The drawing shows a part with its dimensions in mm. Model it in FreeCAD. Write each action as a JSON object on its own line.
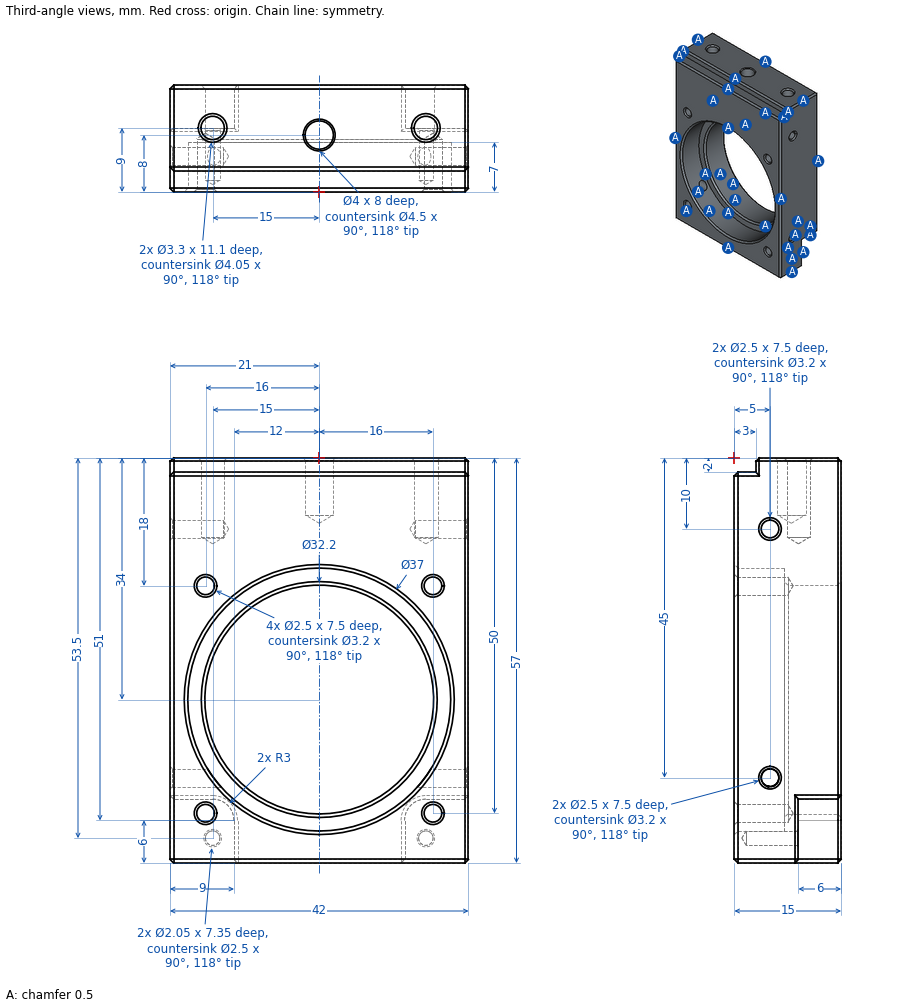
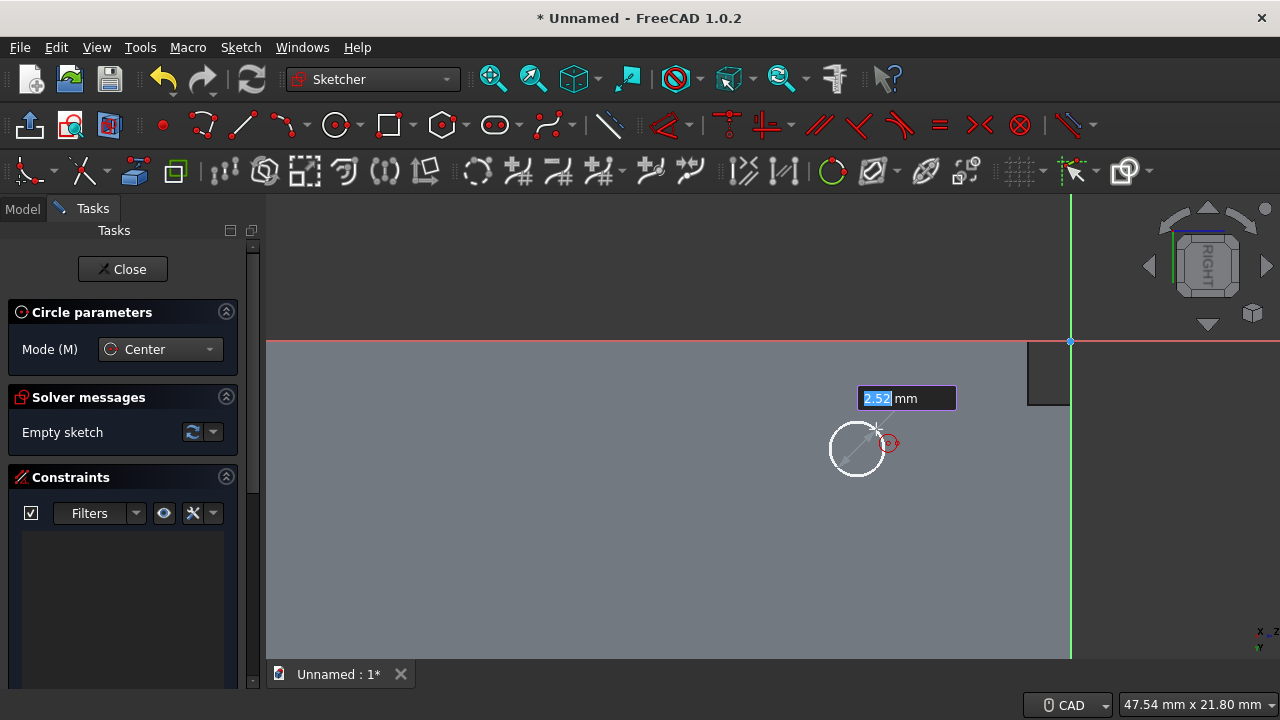
{"action": "type", "text": "2.5"}
{"action": "key", "text": "Return"}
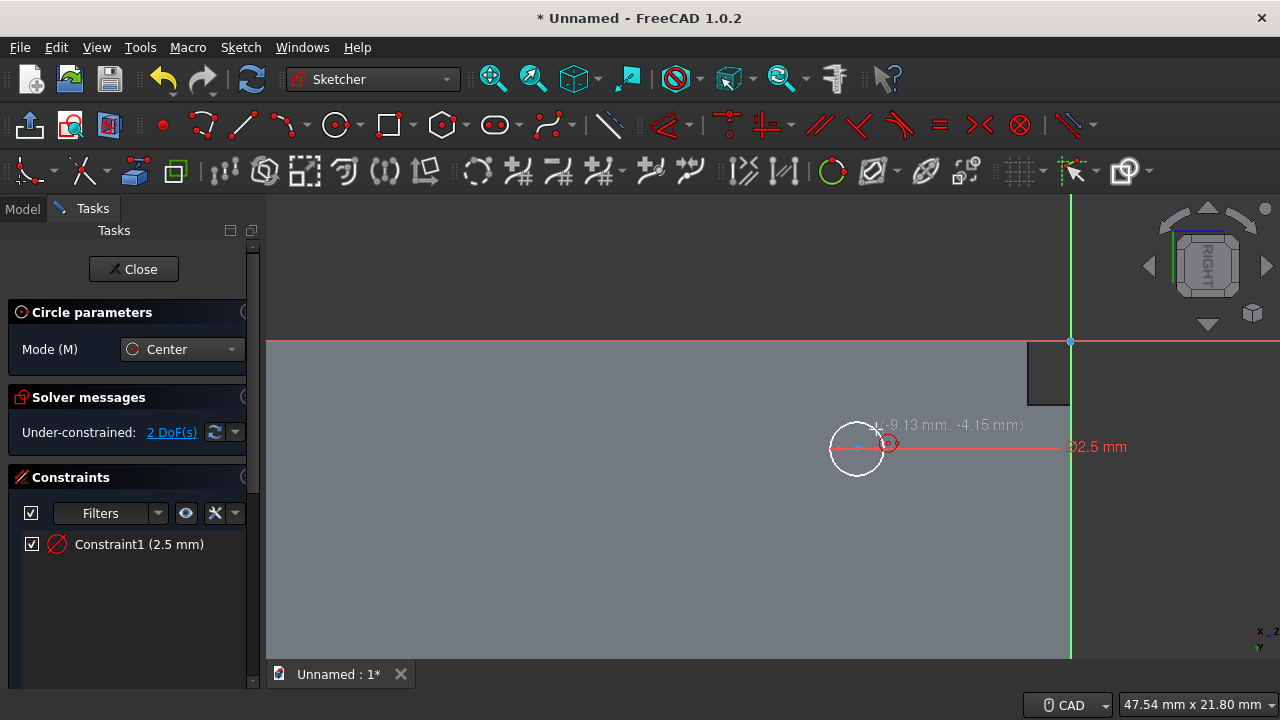
{"action": "scroll", "coordinate": [859, 449], "scroll_direction": "down", "scroll_amount": 3}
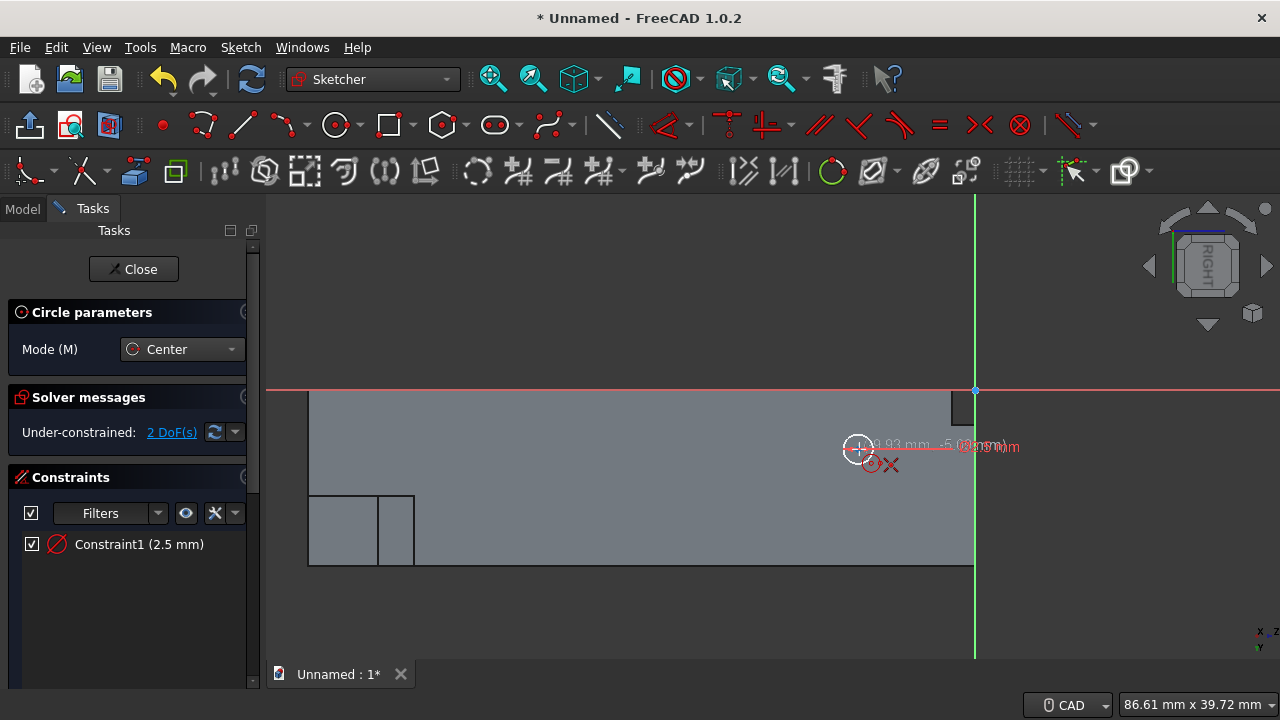
{"action": "scroll", "coordinate": [449, 449], "scroll_direction": "up", "scroll_amount": 3}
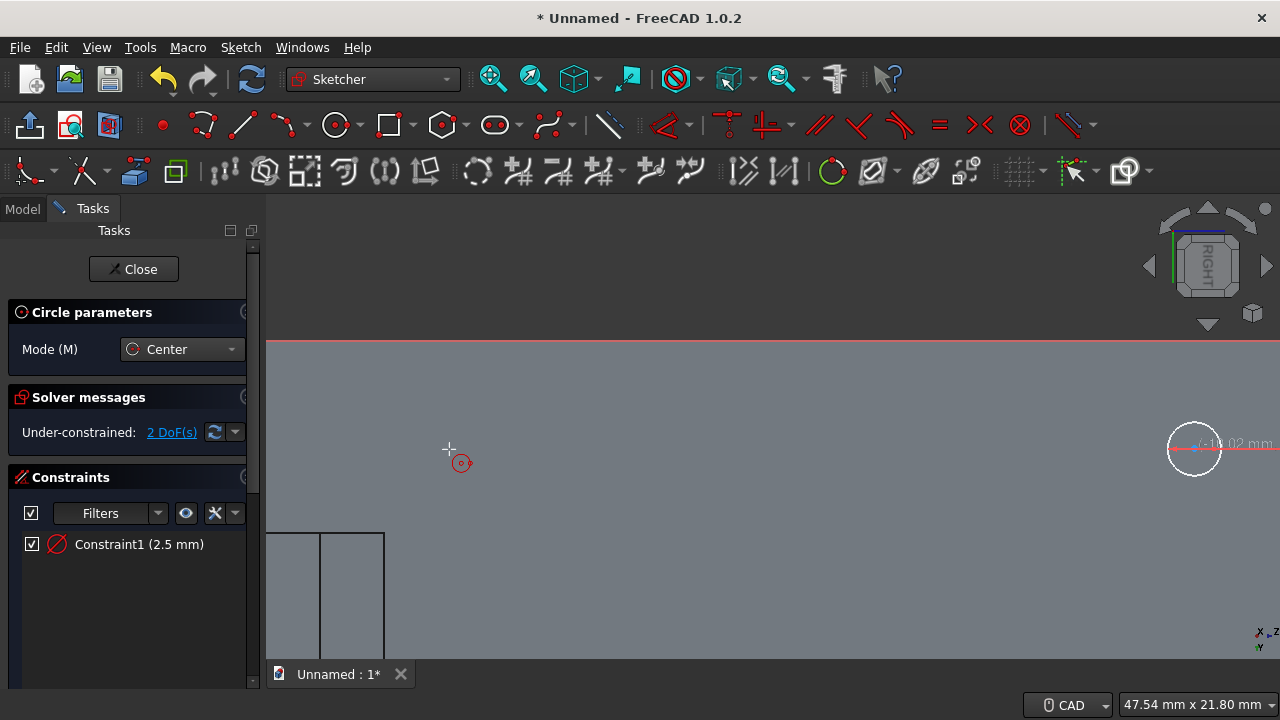
{"action": "left_click", "coordinate": [448, 448]}
{"action": "mouse_move", "coordinate": [467, 429]}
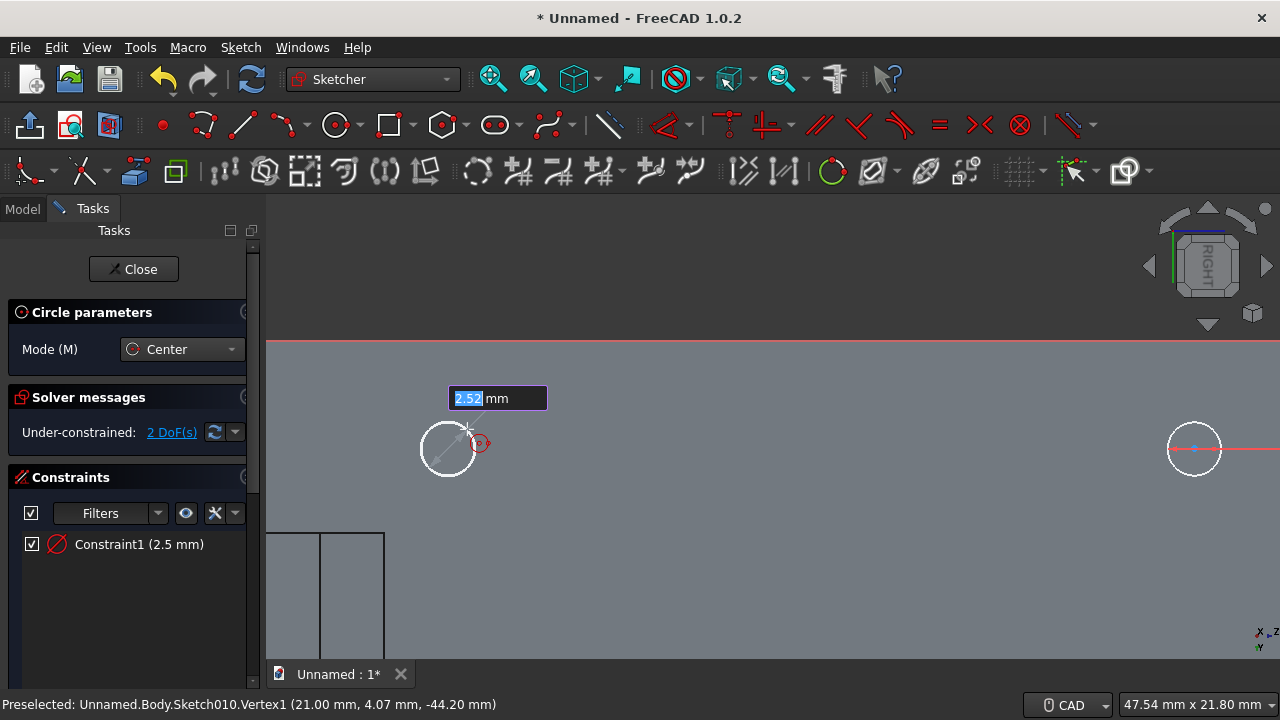
{"action": "type", "text": "2.5"}
{"action": "key", "text": "Return"}
{"action": "key", "text": "Escape"}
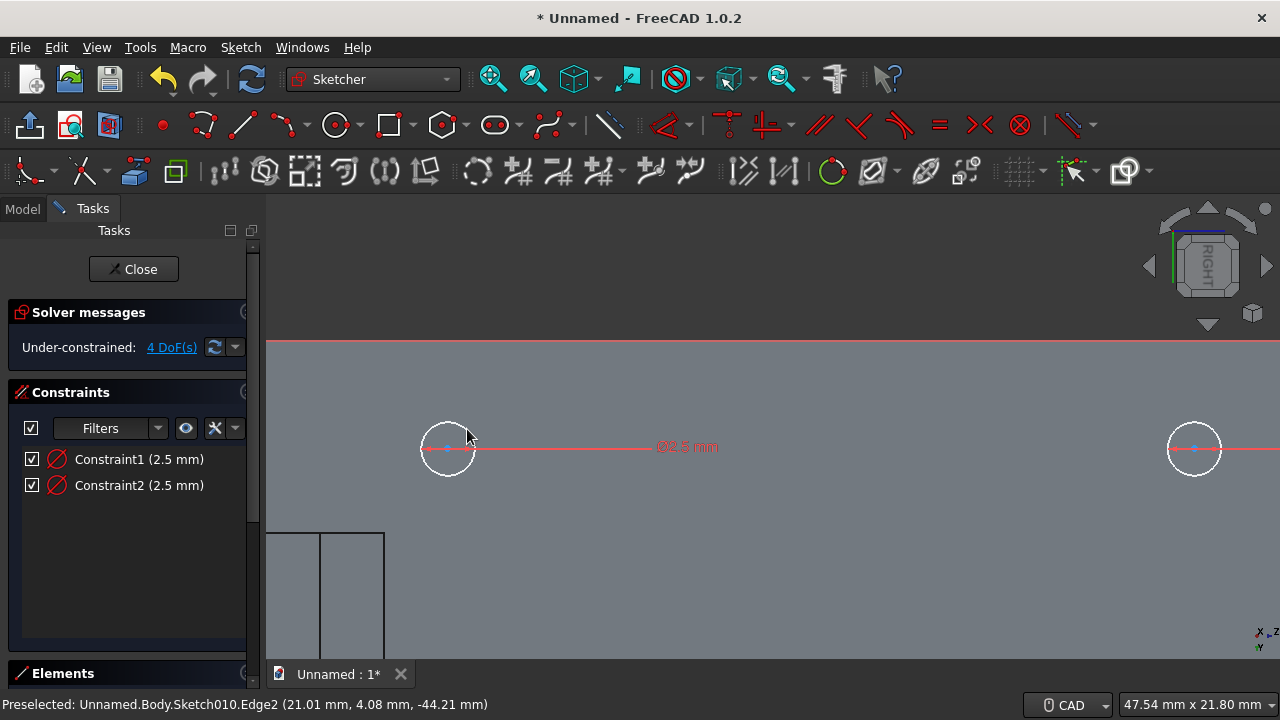
{"action": "key", "text": "d"}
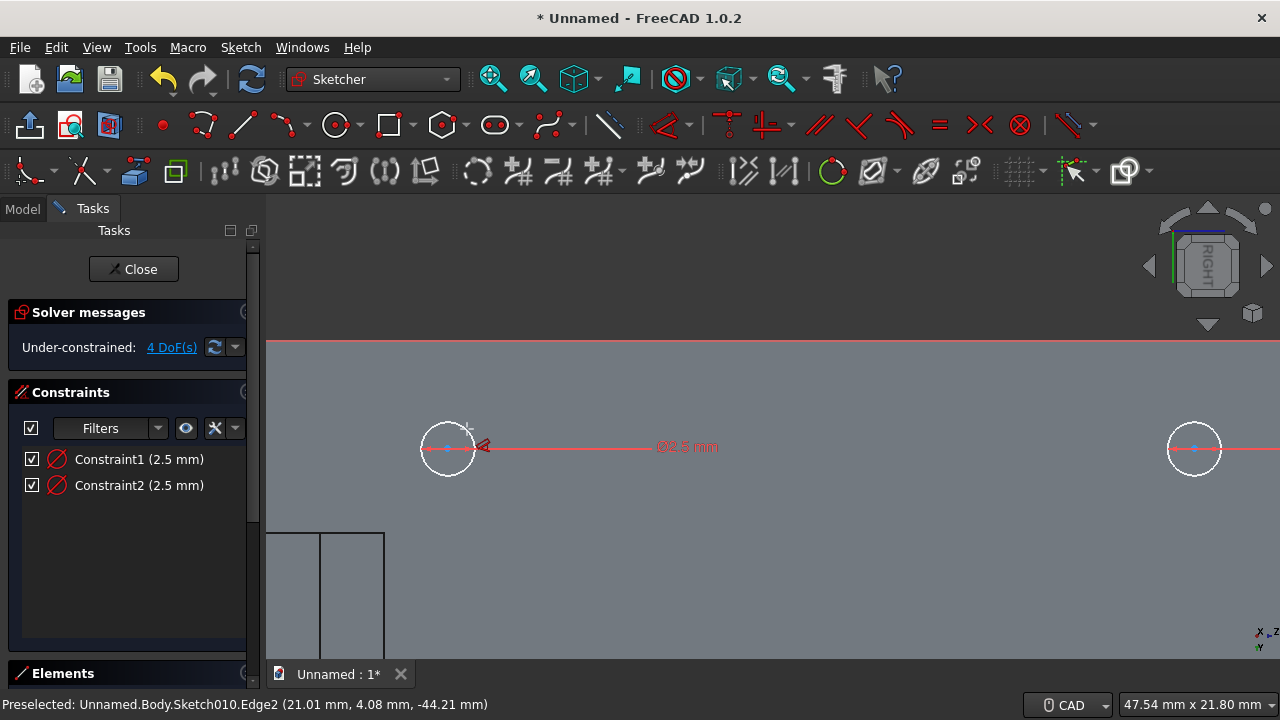
{"action": "scroll", "coordinate": [449, 449], "scroll_direction": "down", "scroll_amount": 3}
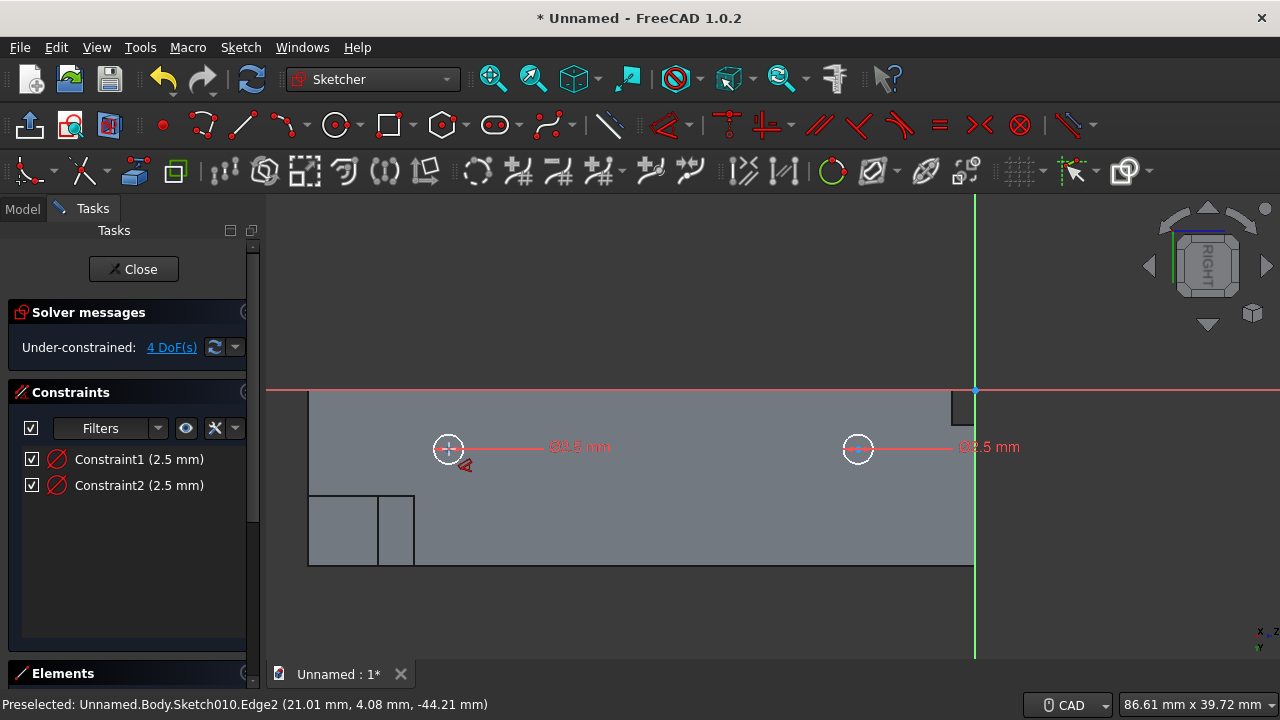
{"action": "left_click", "coordinate": [858, 449]}
{"action": "left_click", "coordinate": [1009, 420]}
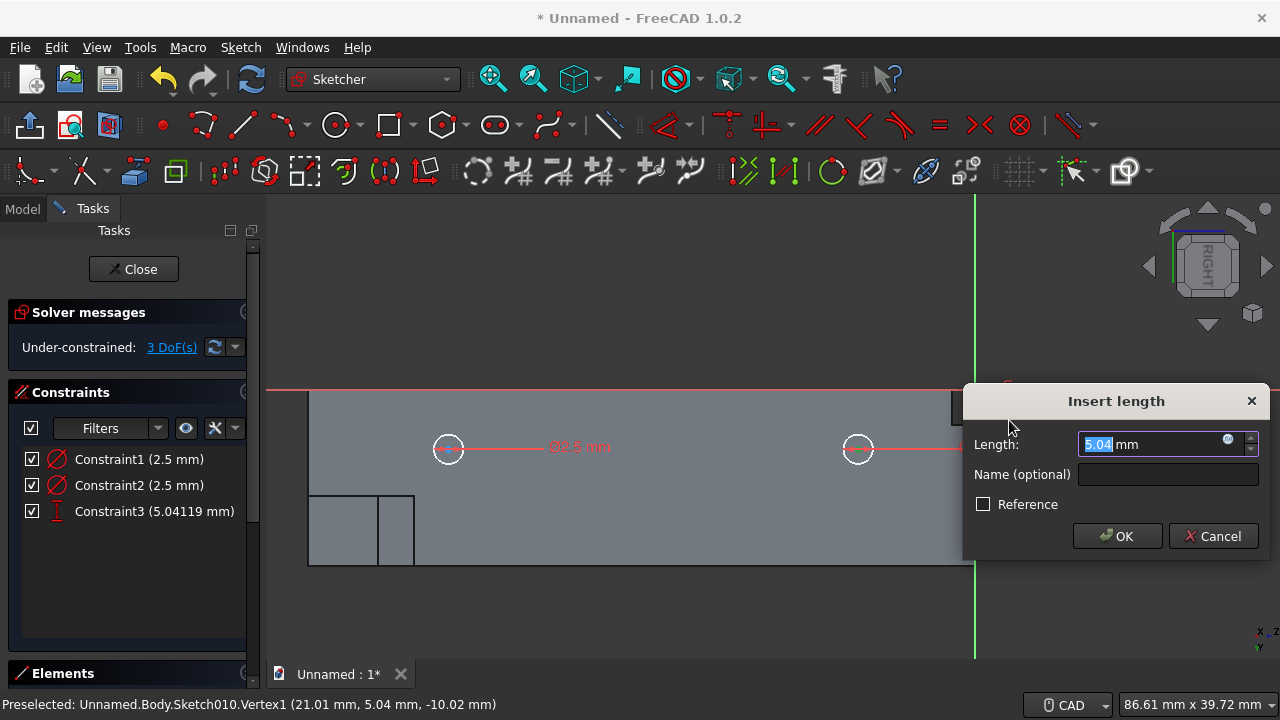
{"action": "type", "text": "5"}
{"action": "key", "text": "Return"}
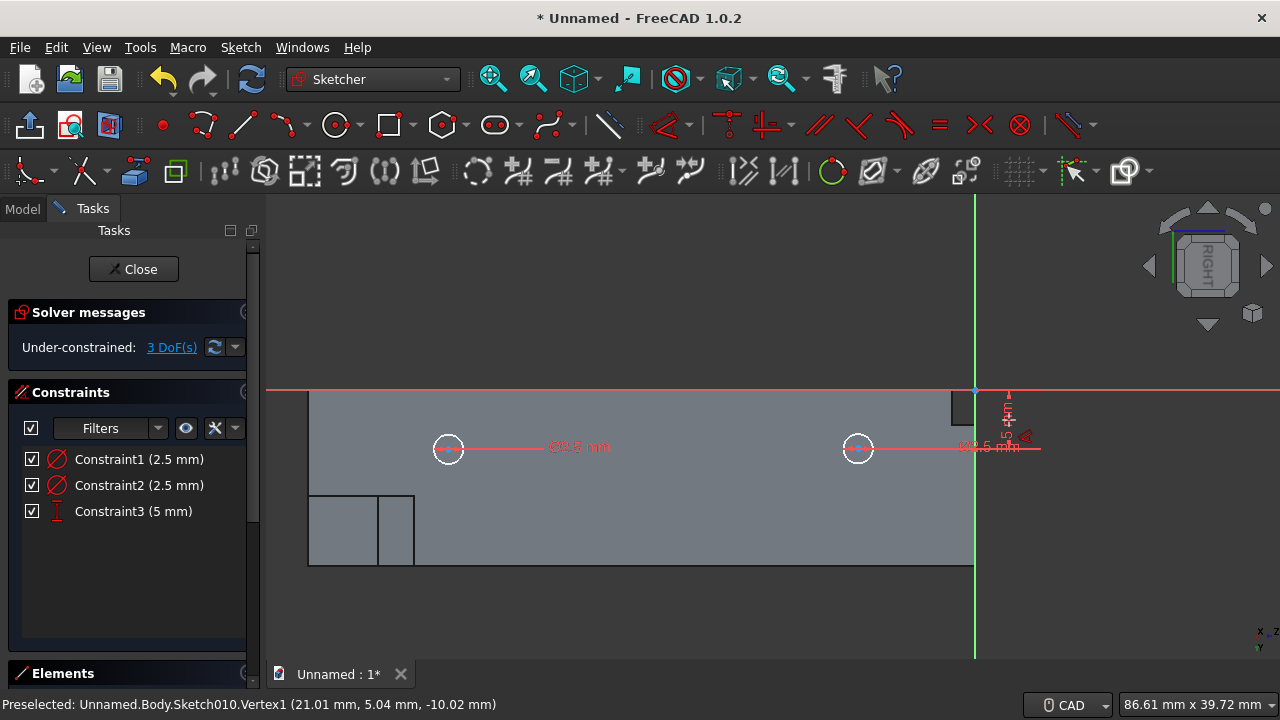
{"action": "left_click", "coordinate": [449, 449]}
{"action": "left_click", "coordinate": [1009, 440]}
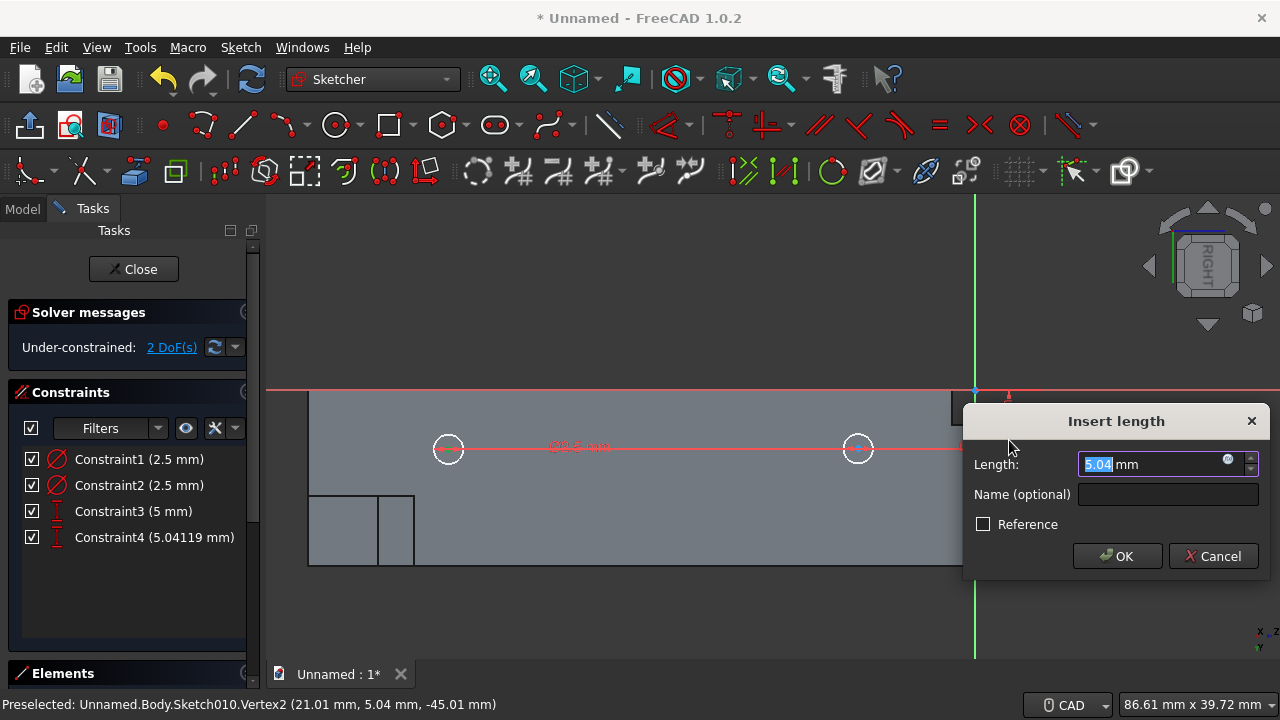
{"action": "type", "text": "5"}
{"action": "key", "text": "Return"}